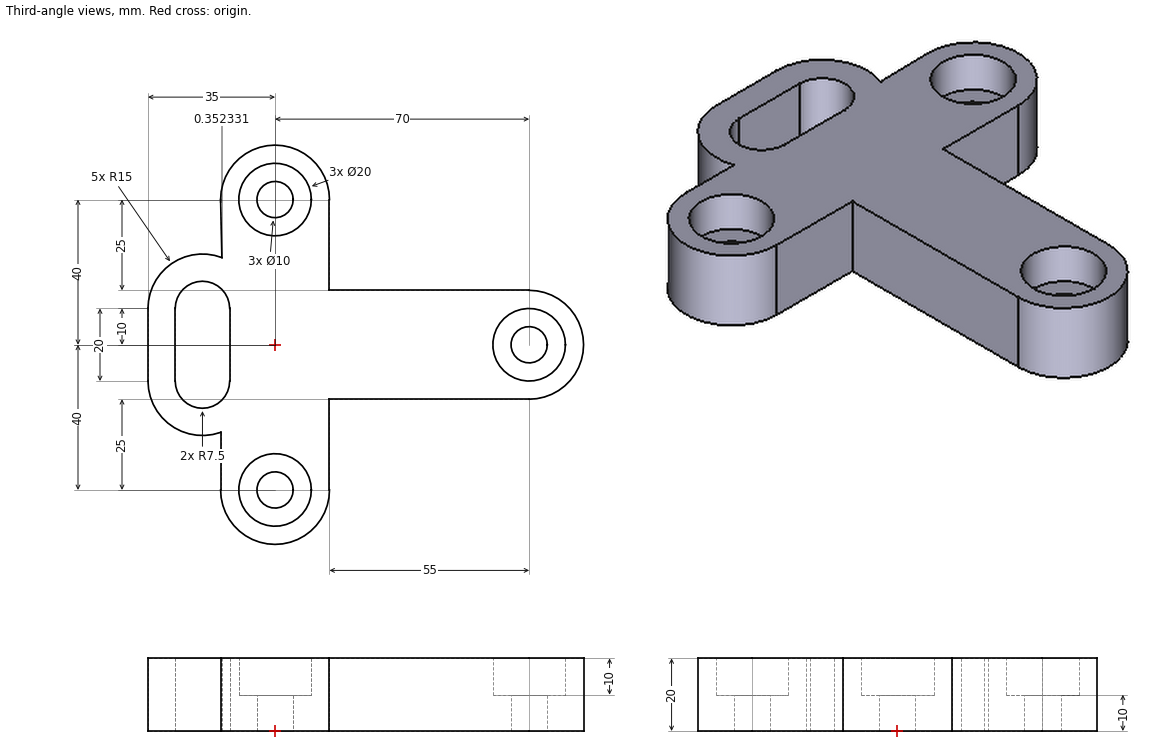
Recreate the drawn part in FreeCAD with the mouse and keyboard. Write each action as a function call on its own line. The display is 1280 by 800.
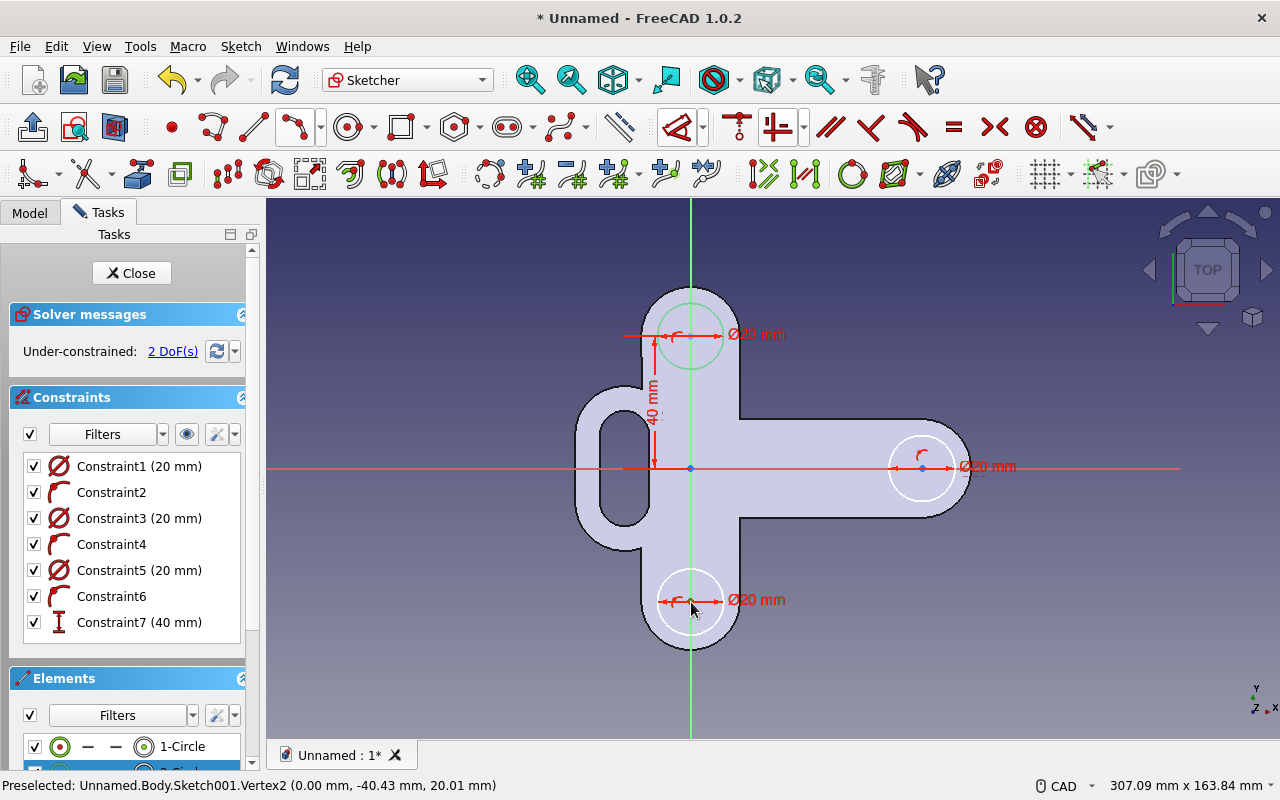
click(702, 128)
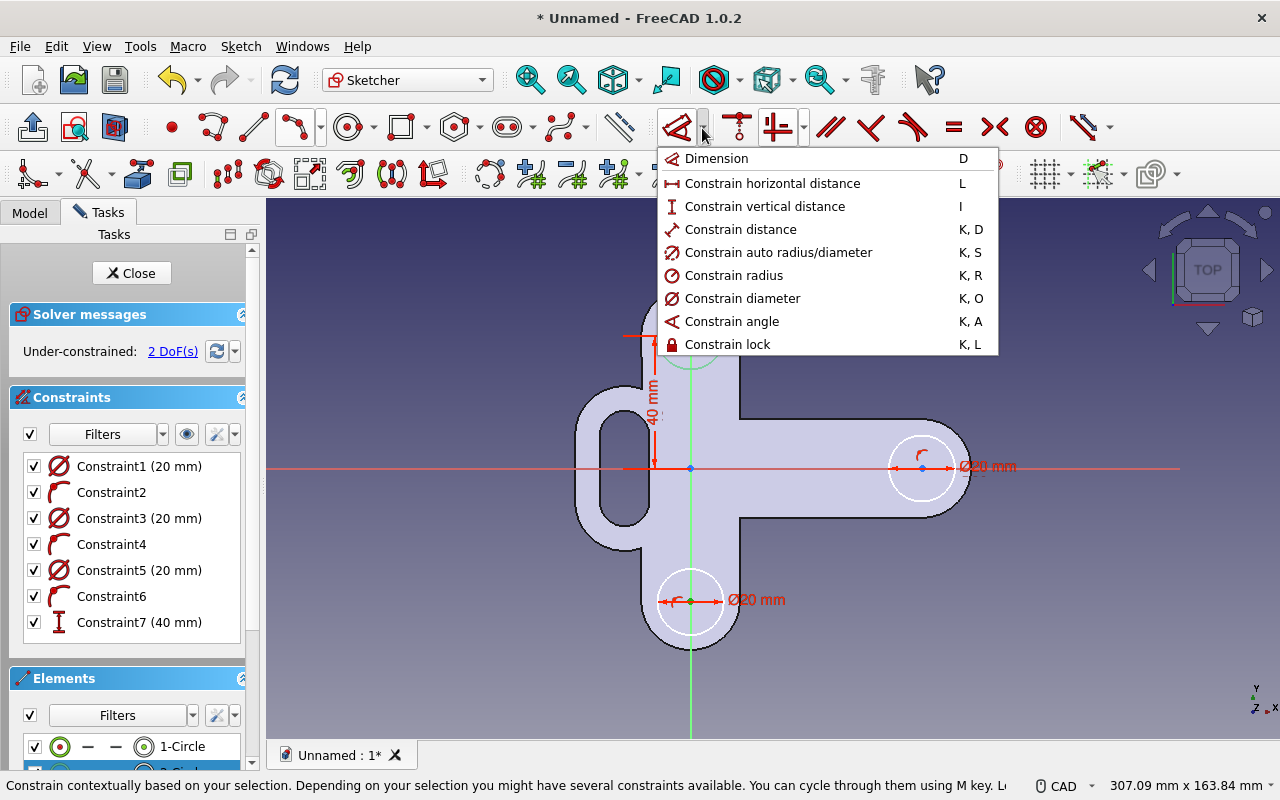
click(828, 206)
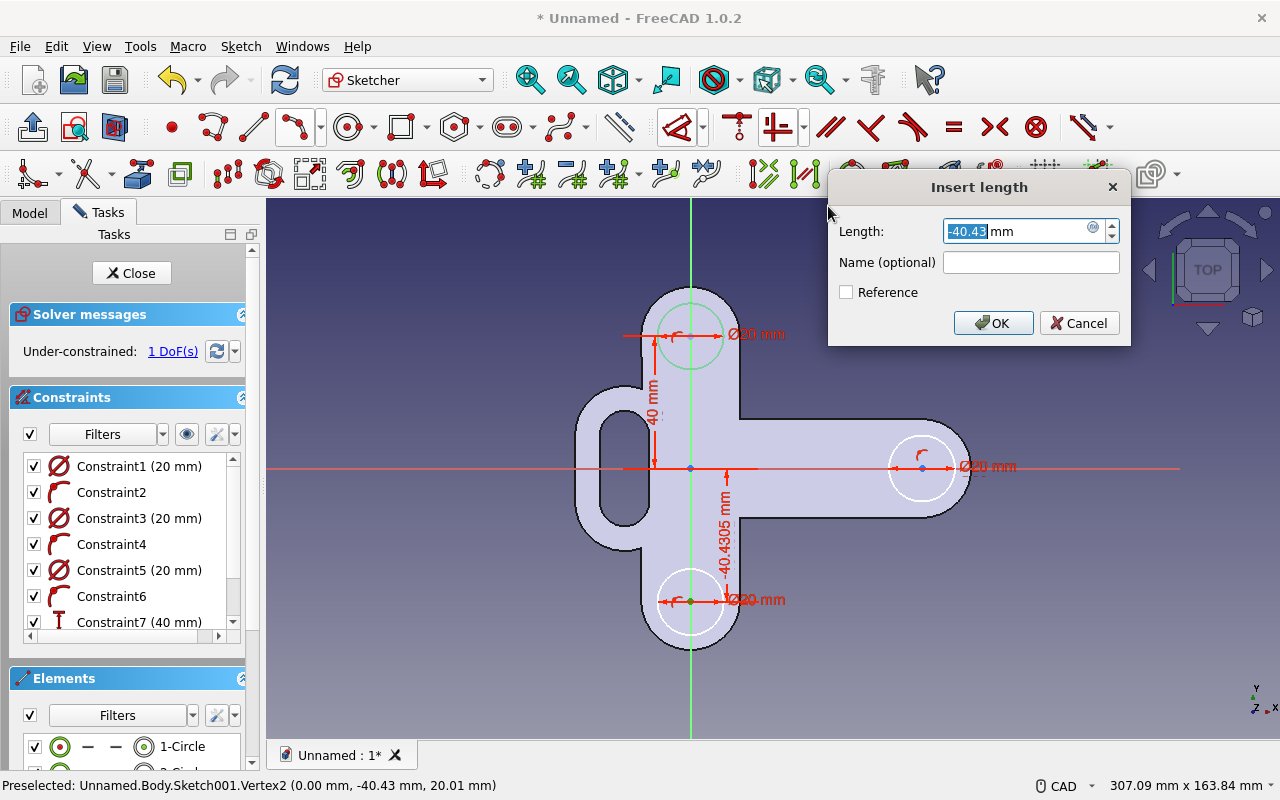
text(-40)
key(Return)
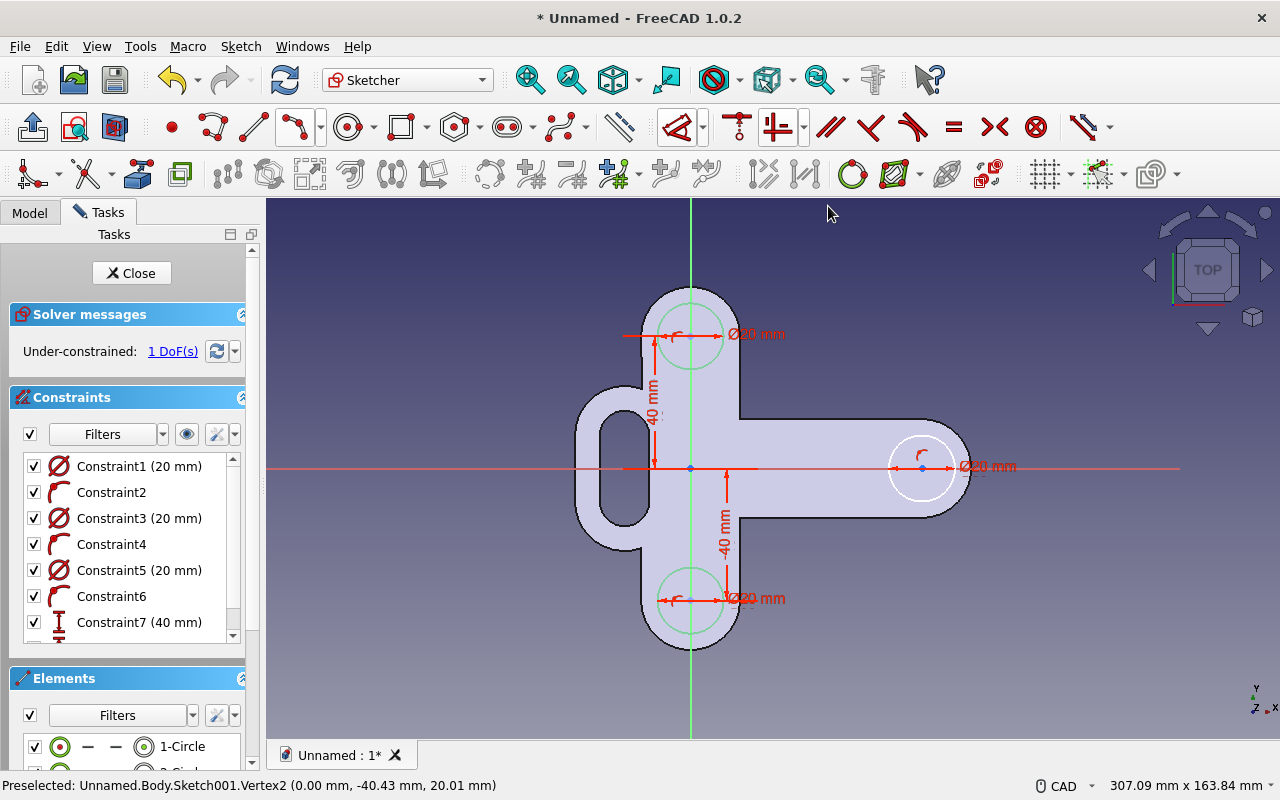
click(922, 468)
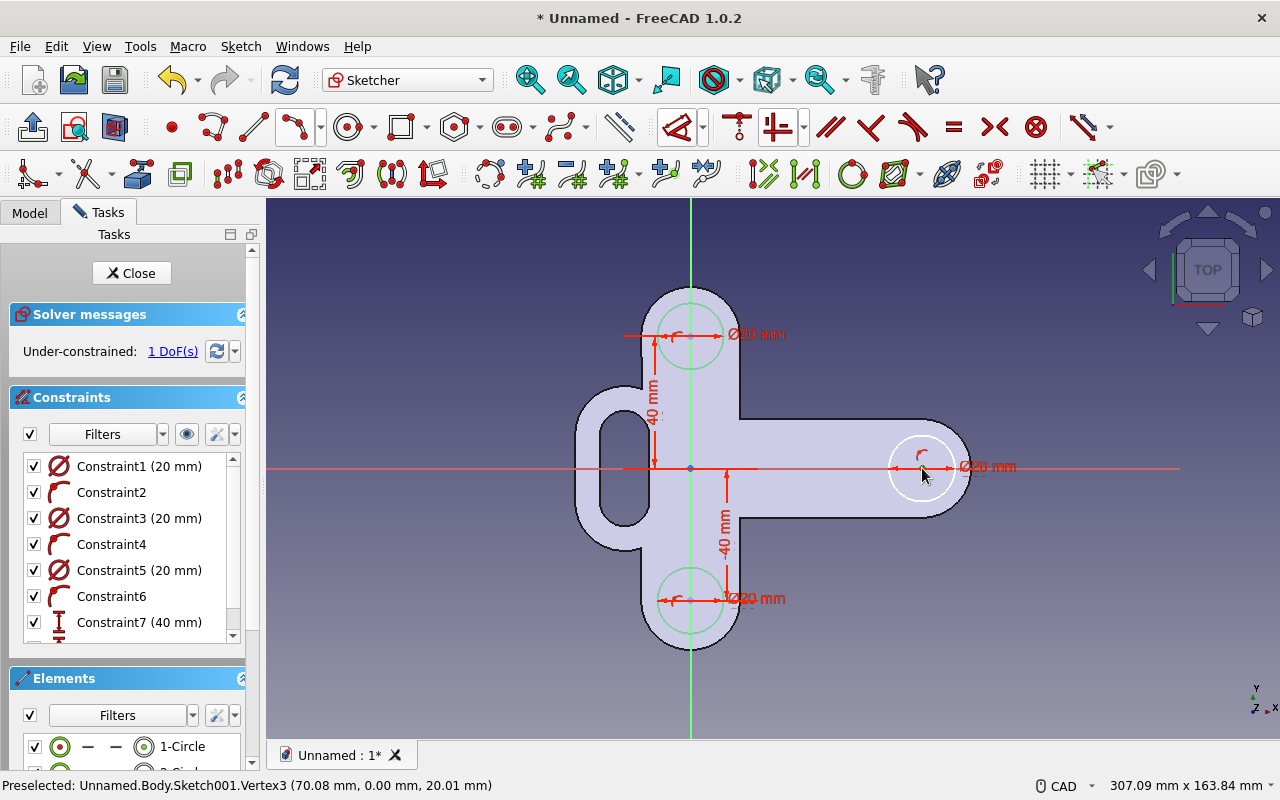
click(702, 128)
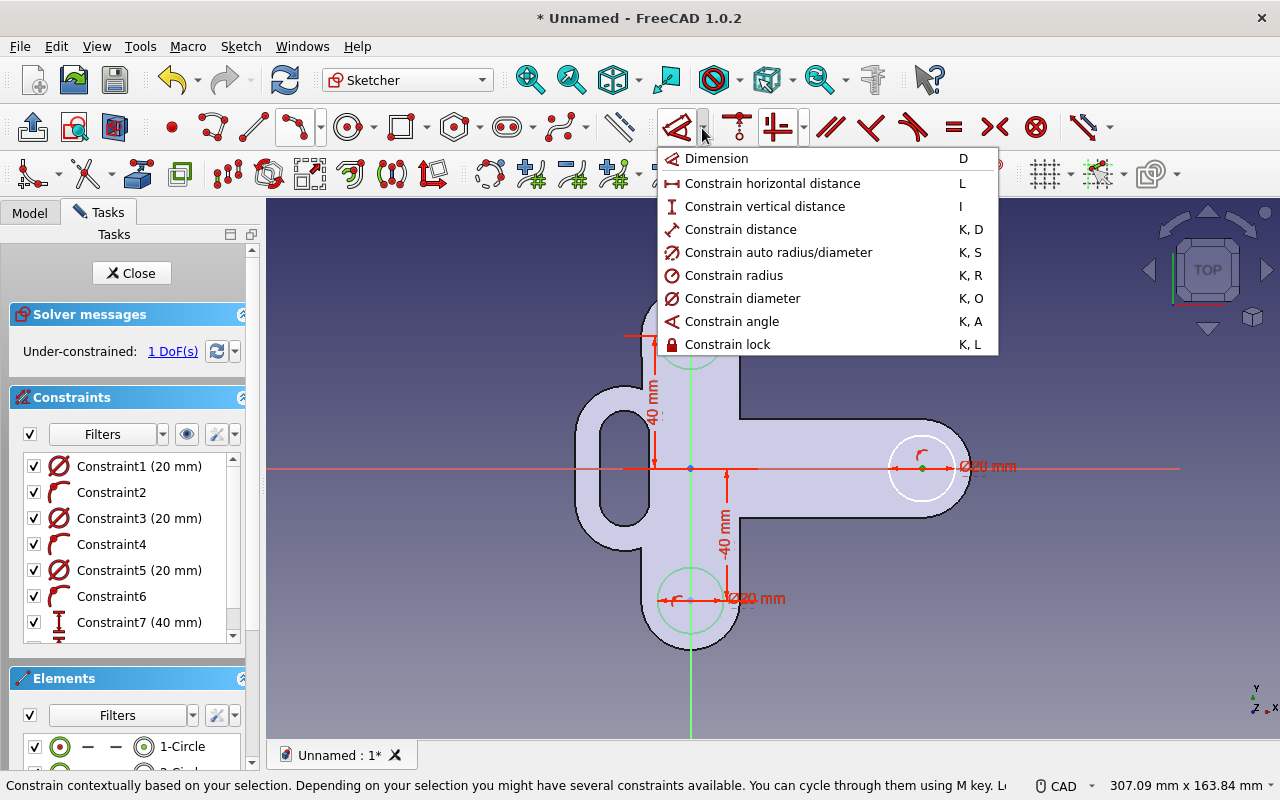
click(828, 184)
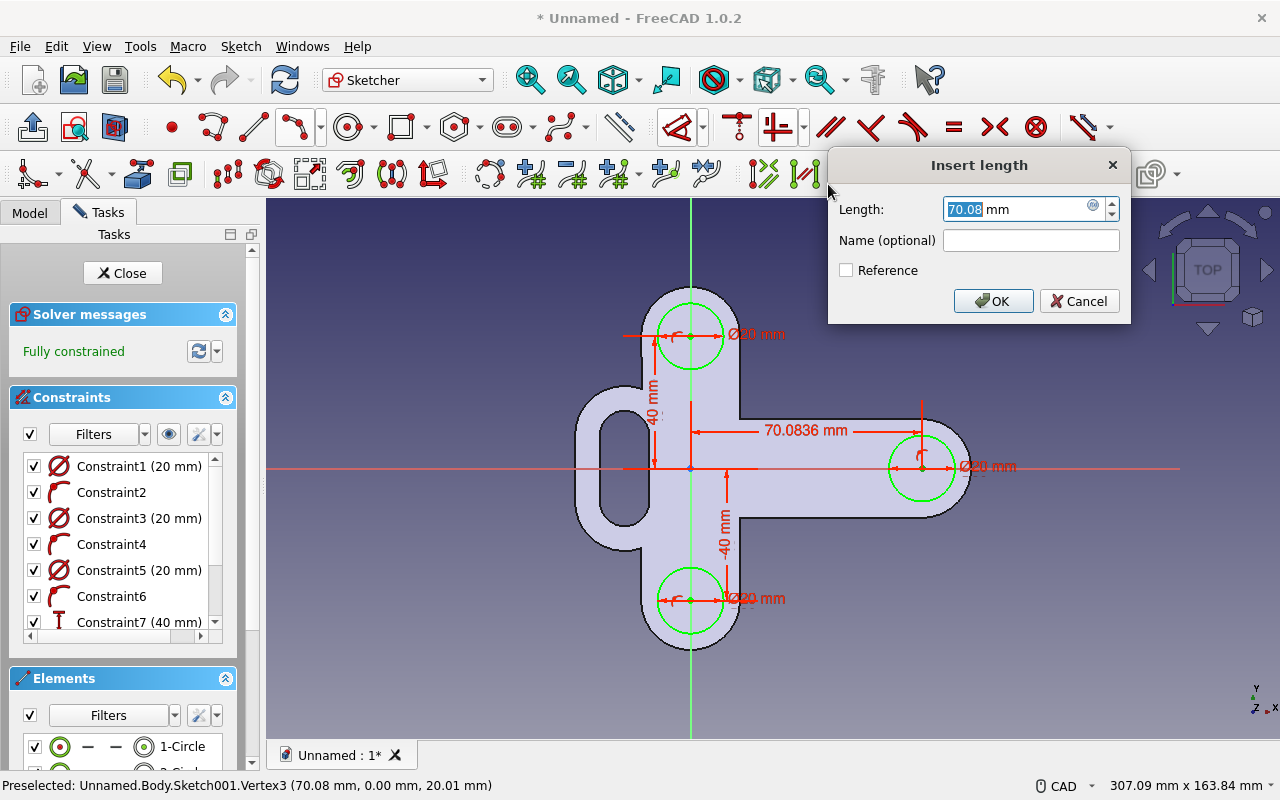
text(70)
key(Return)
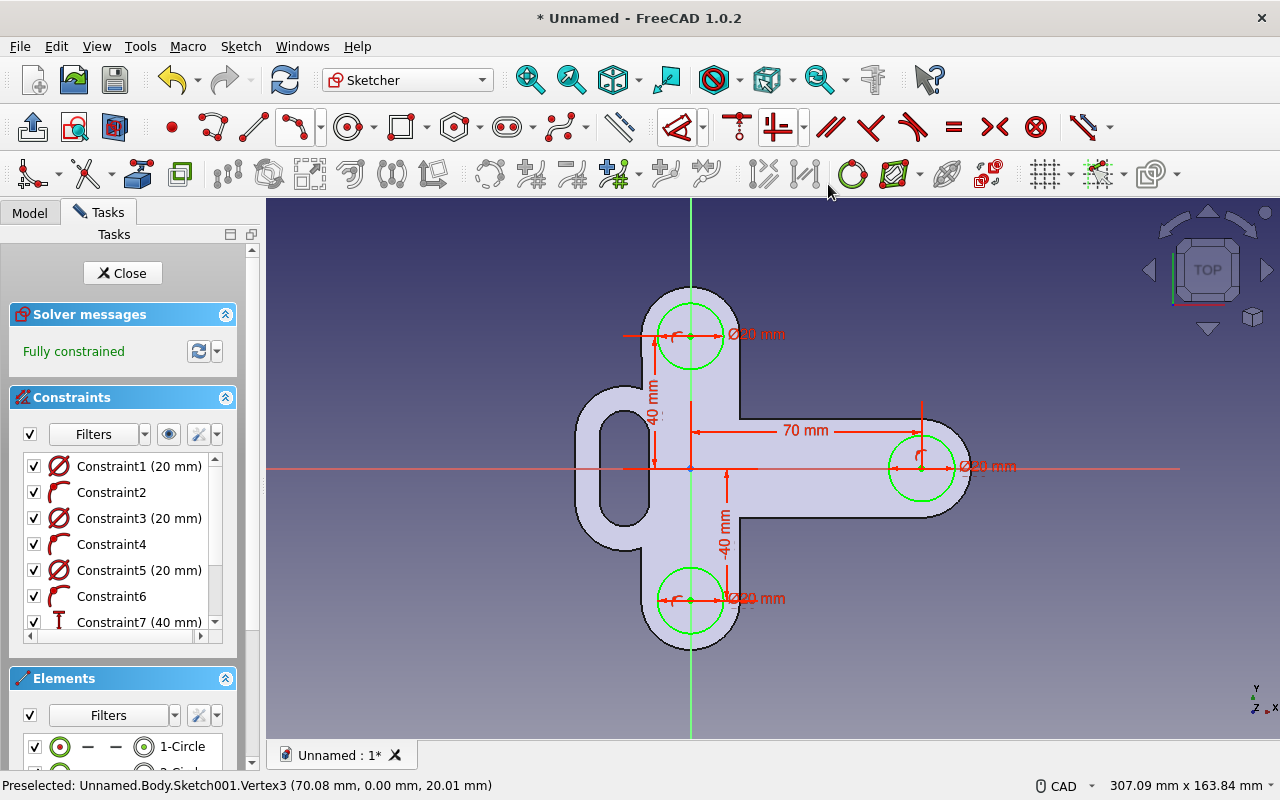
click(123, 273)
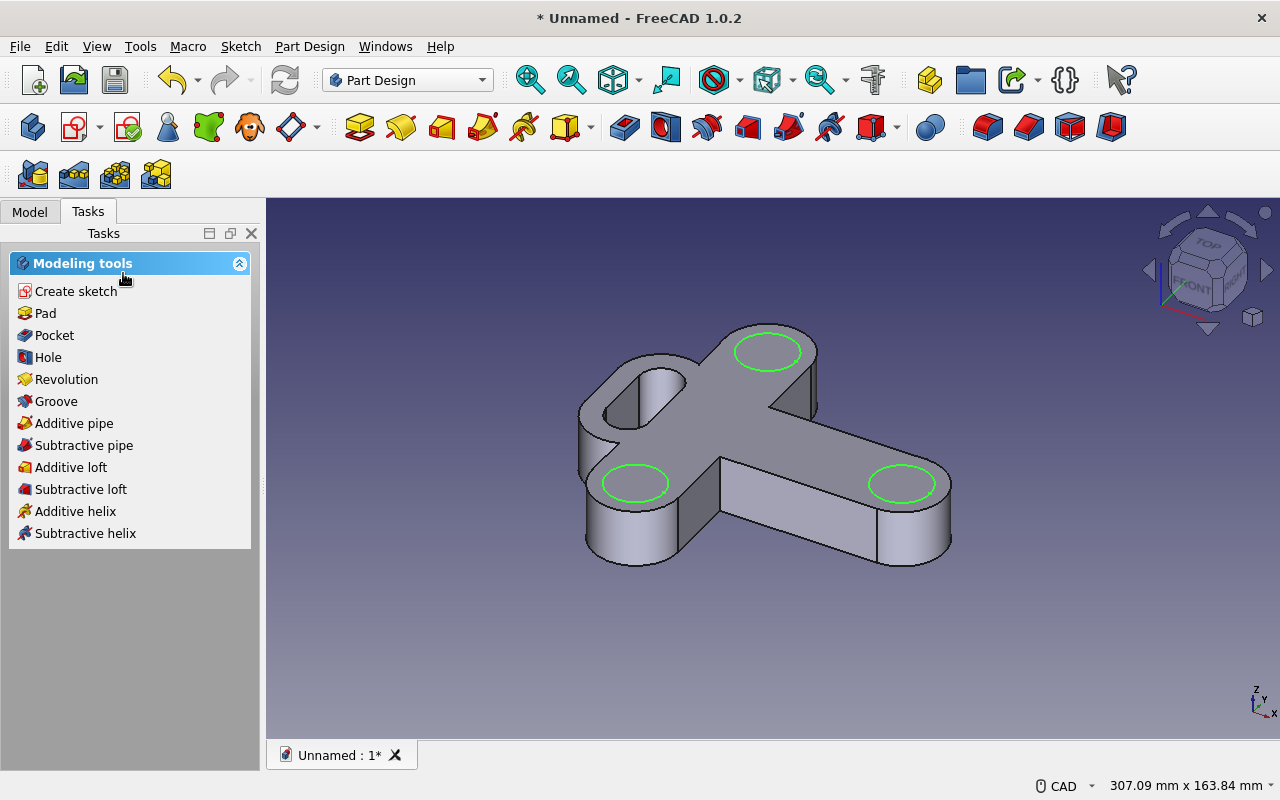
click(625, 128)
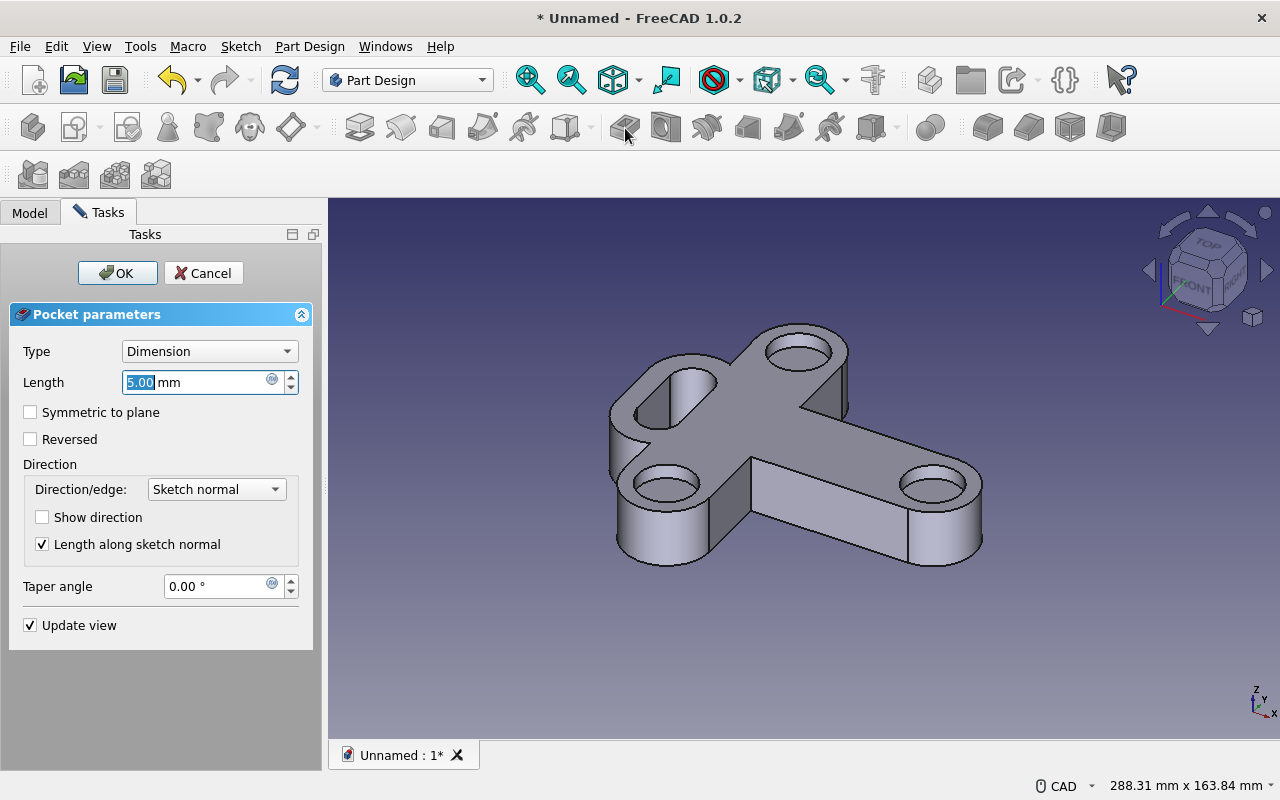
text(10)
key(Tab)